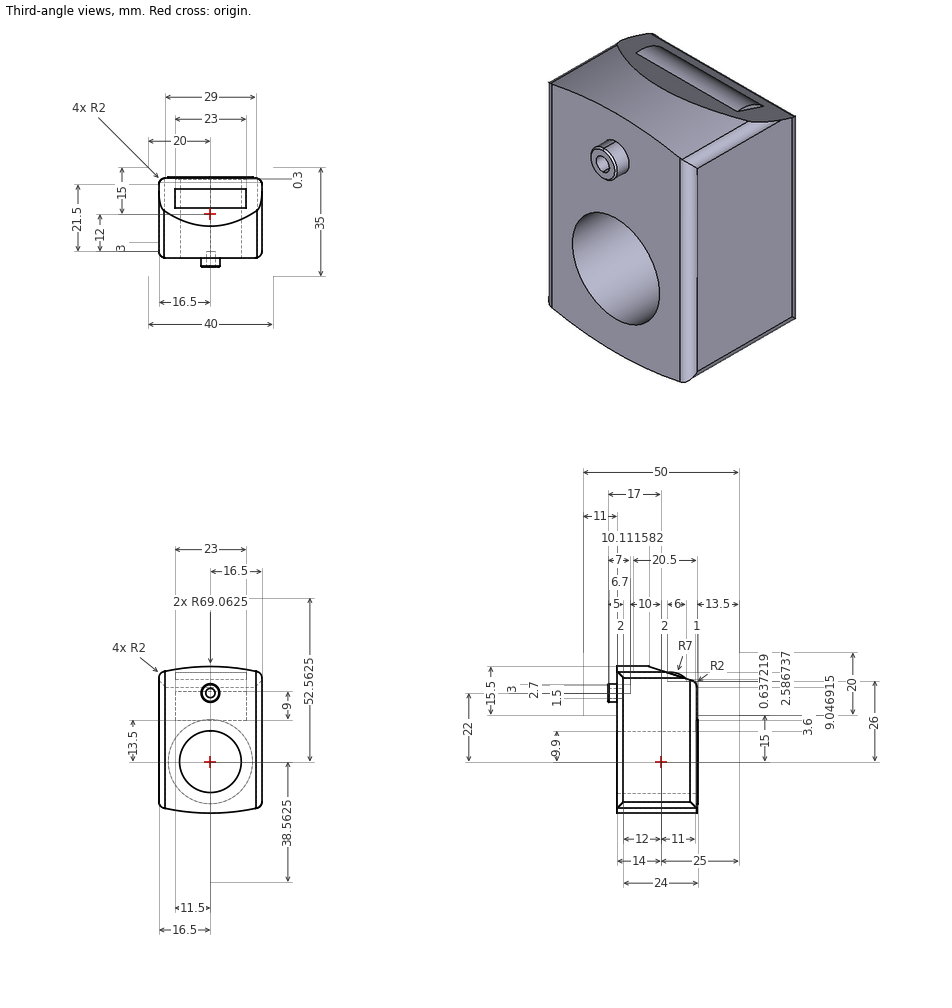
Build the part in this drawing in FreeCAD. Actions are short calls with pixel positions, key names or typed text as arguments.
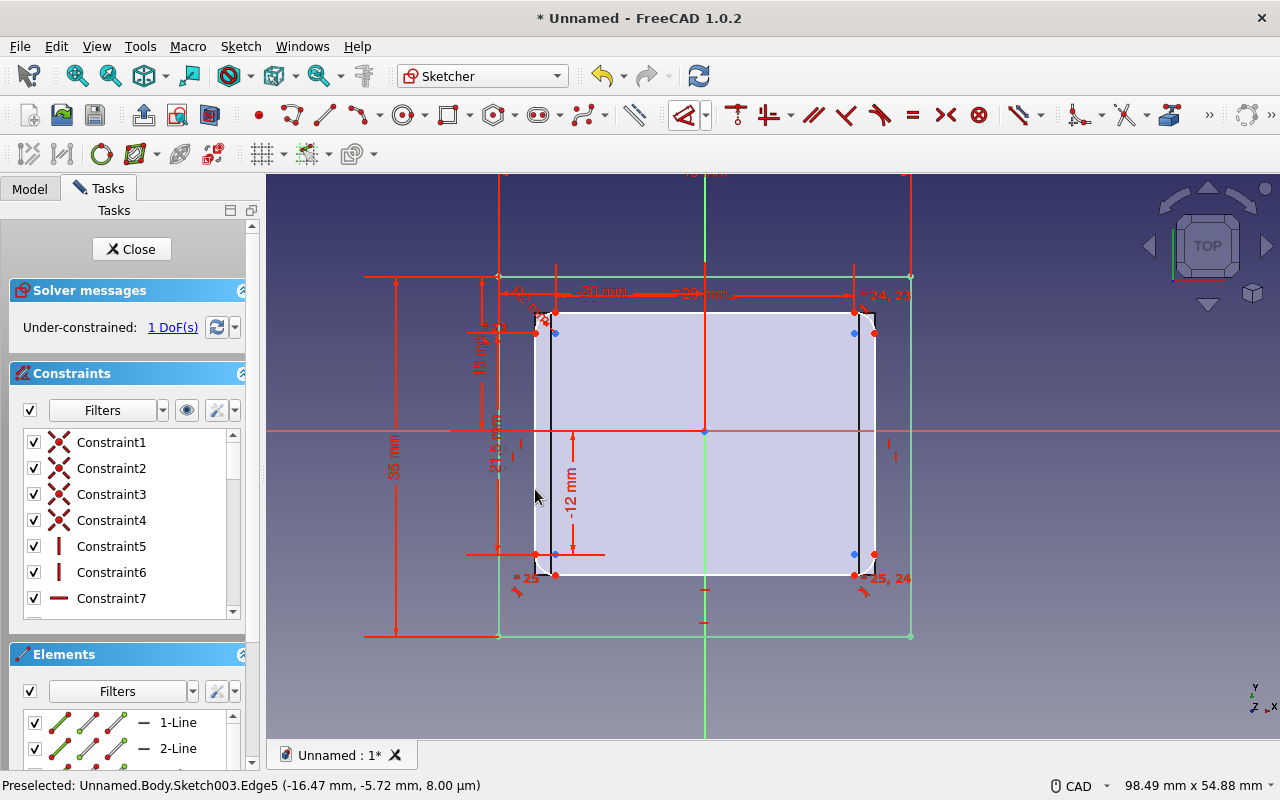
click(535, 555)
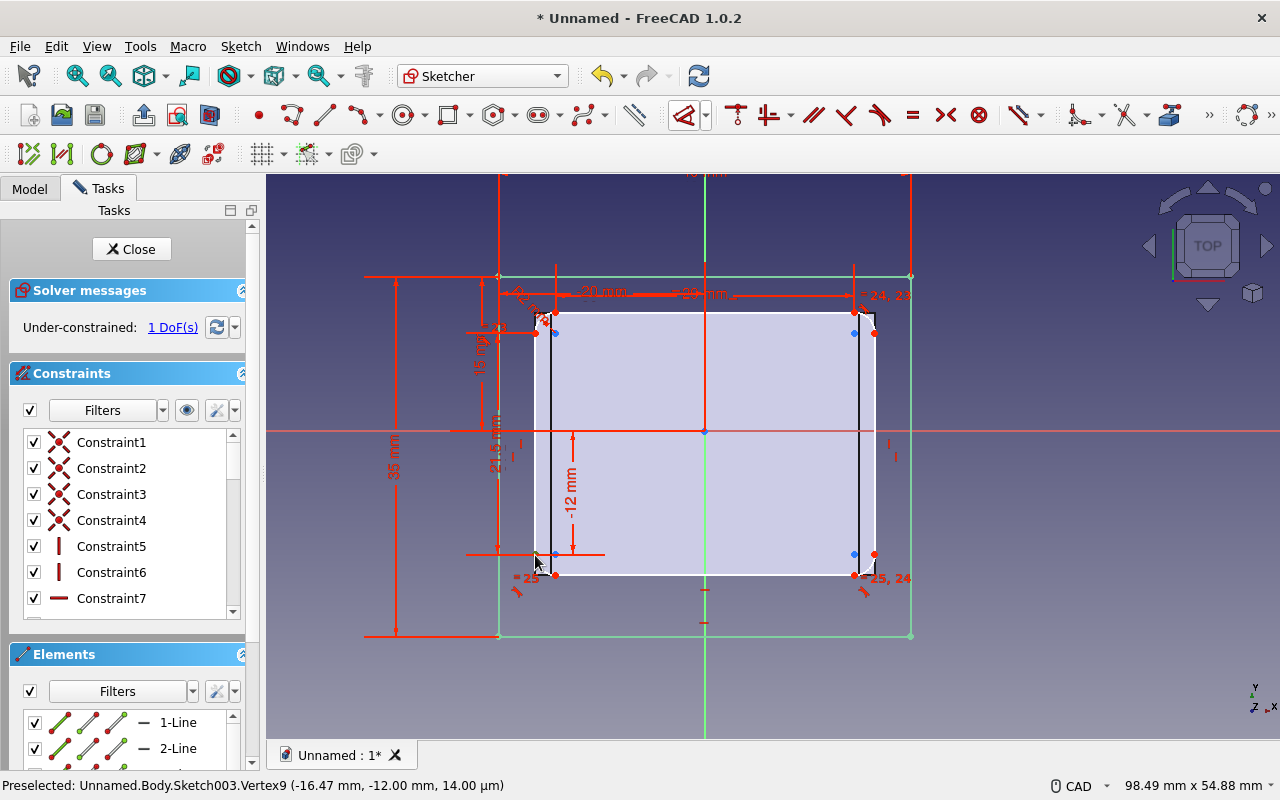
click(706, 116)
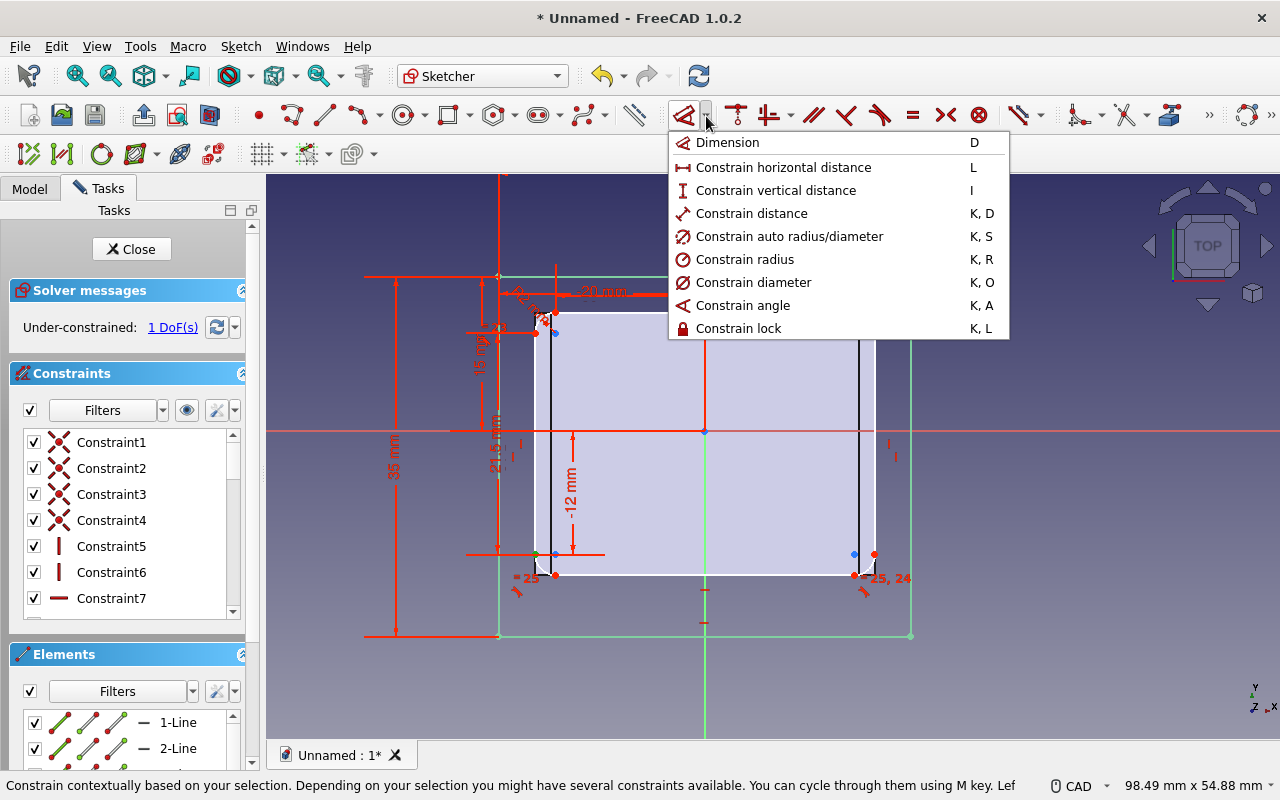
click(839, 168)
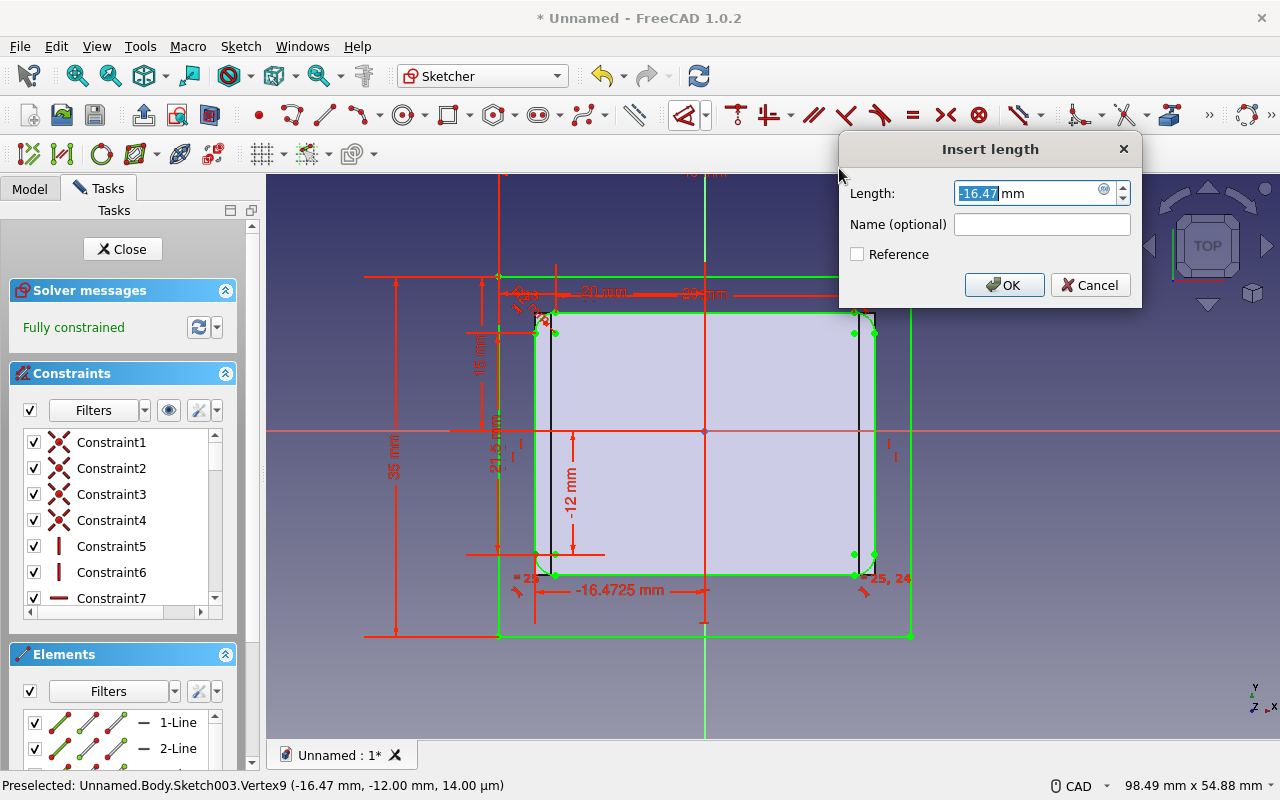
text(-16.5)
key(Return)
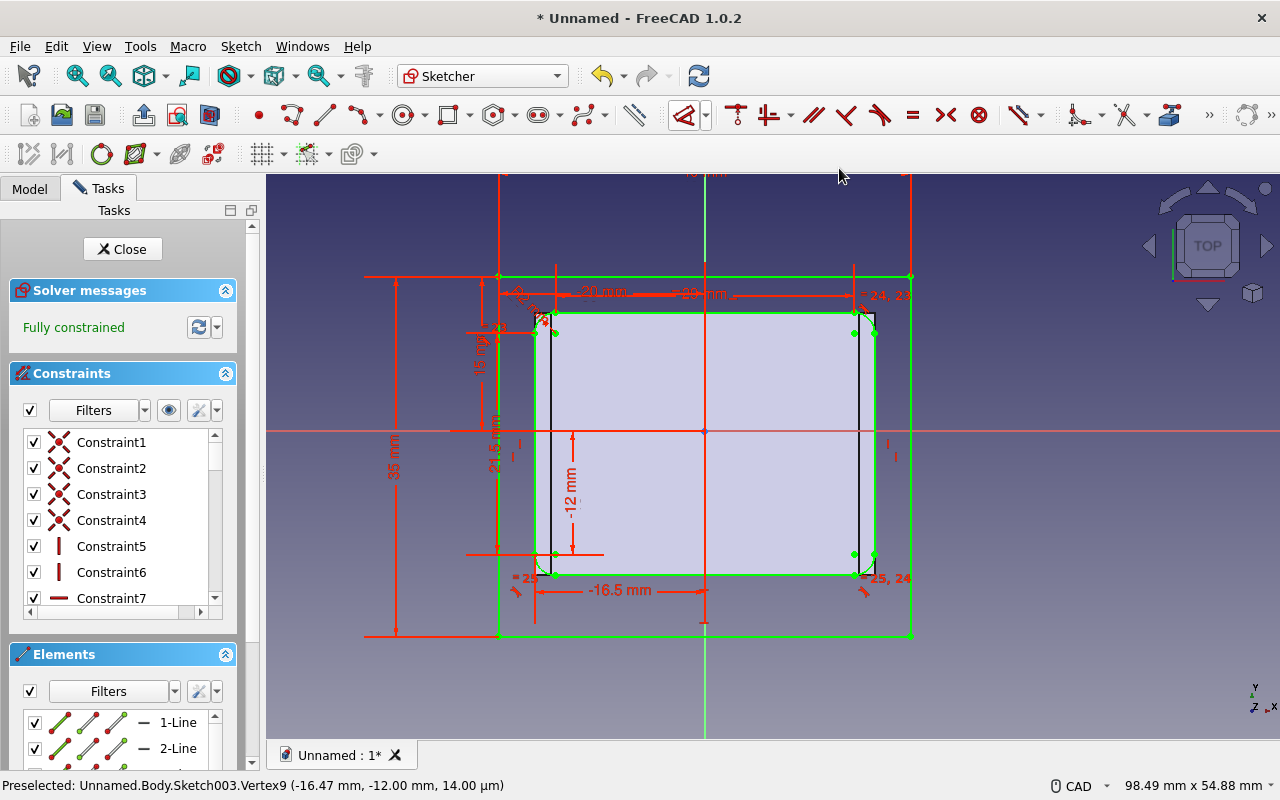
click(123, 249)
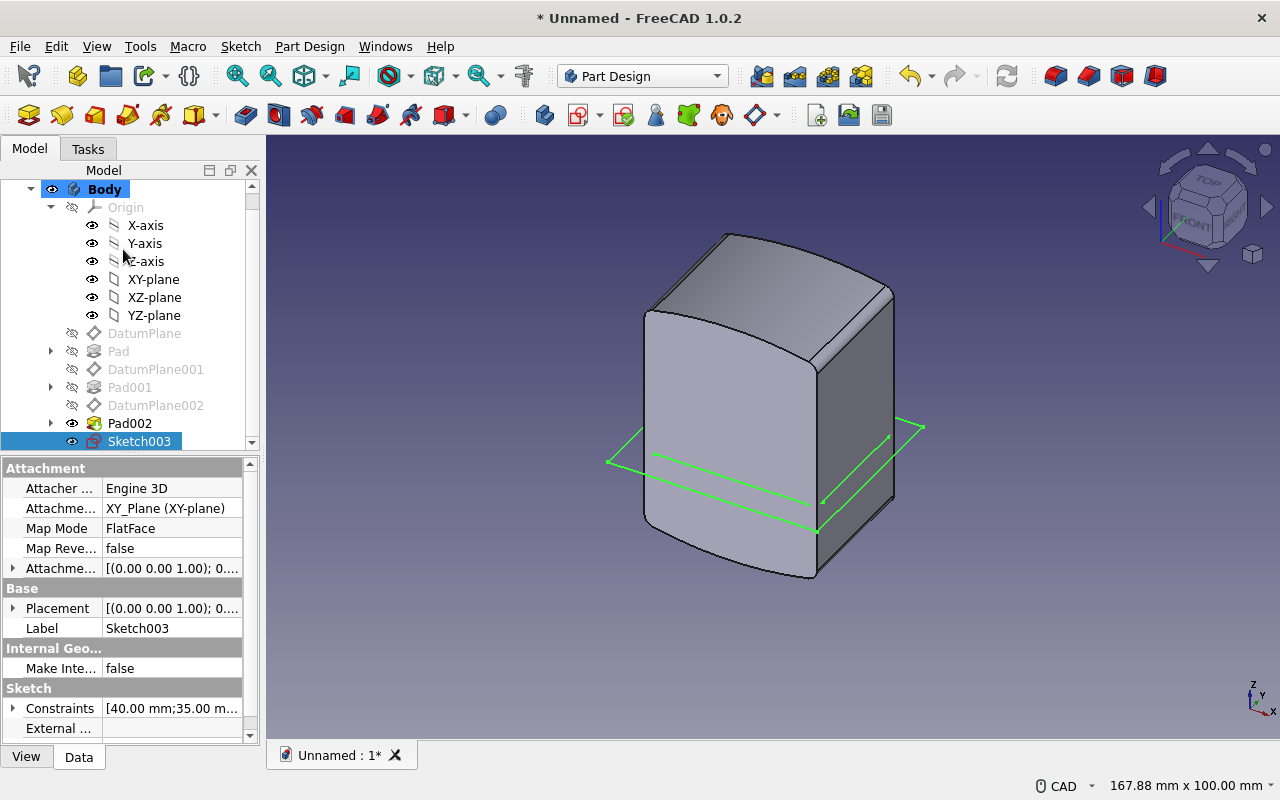
click(246, 116)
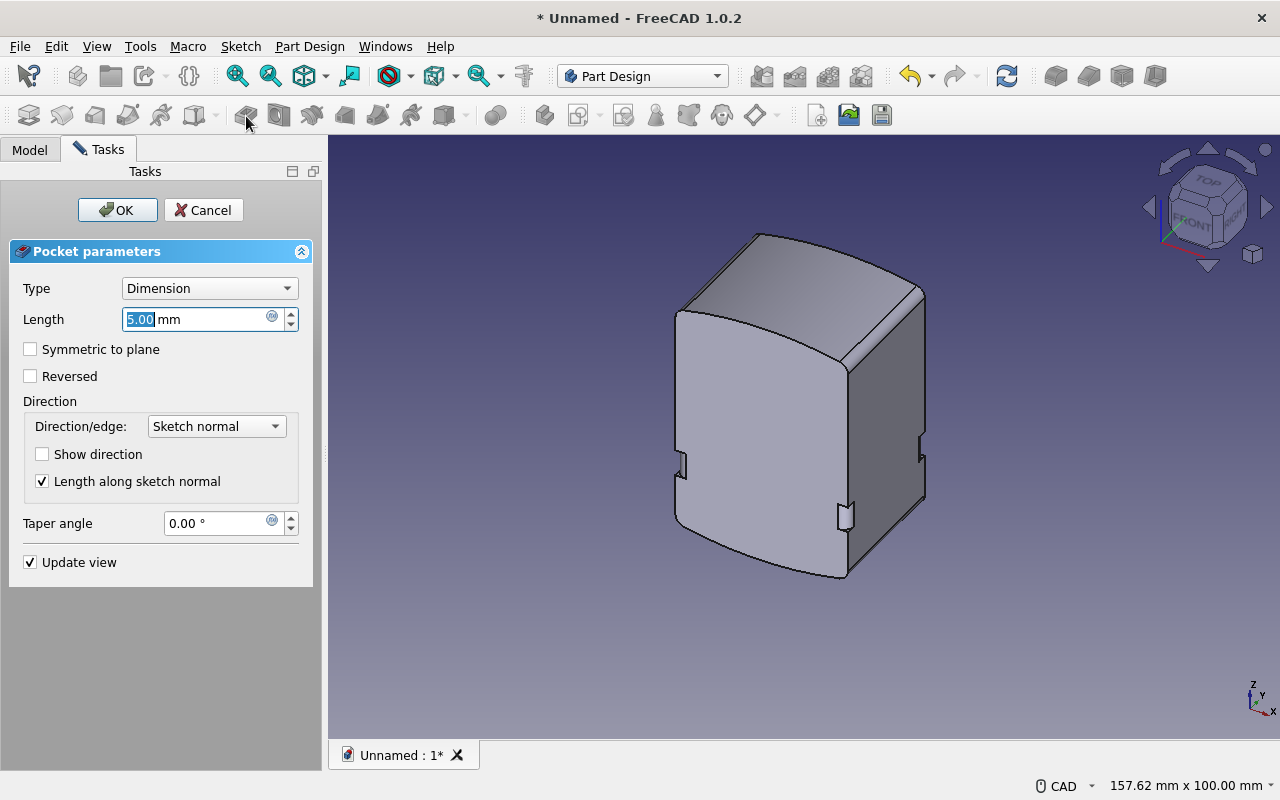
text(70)
key(Tab)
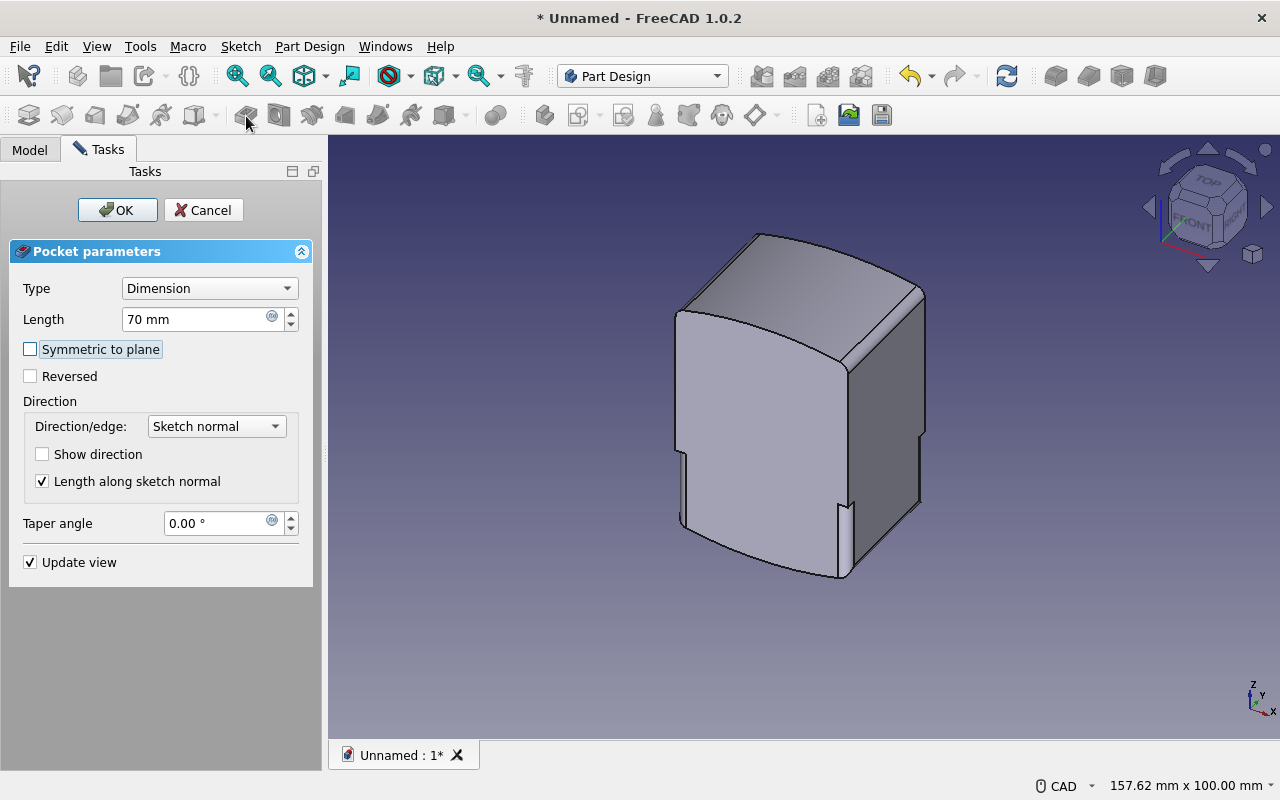
click(31, 349)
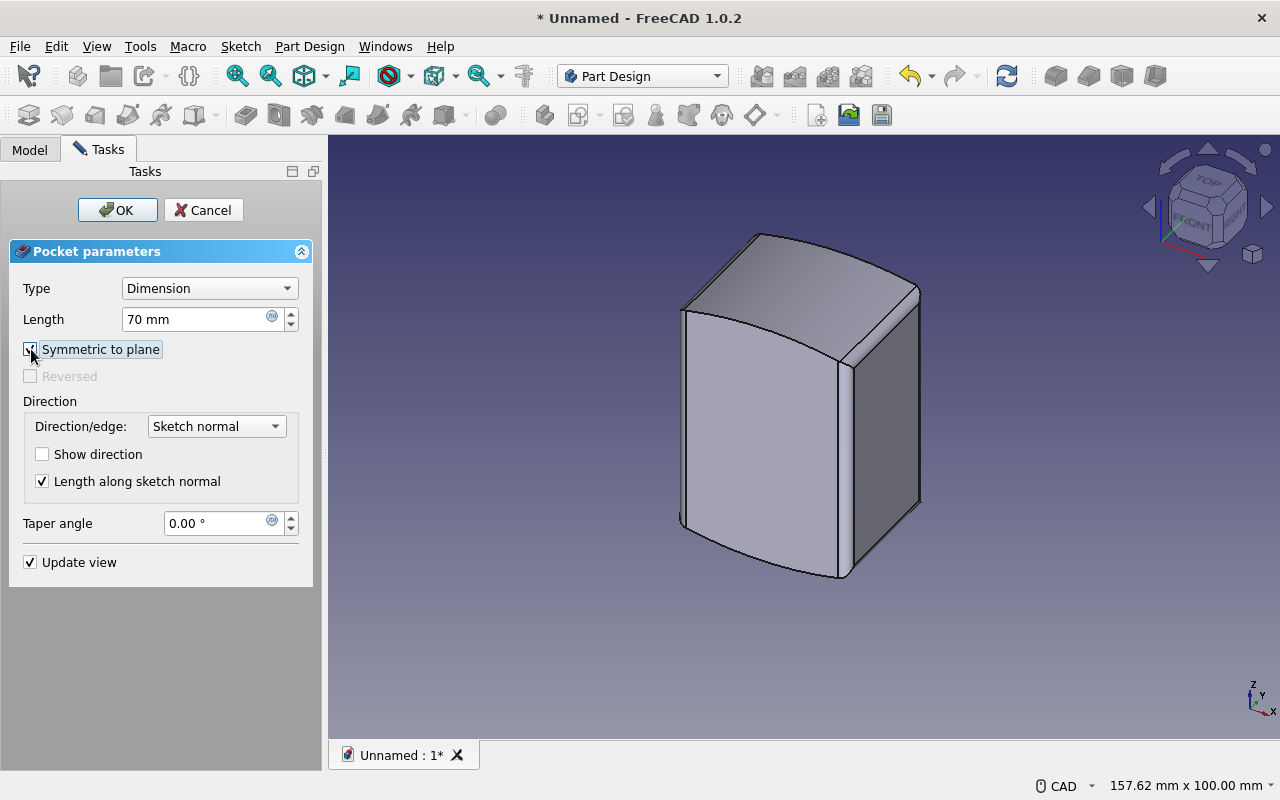
click(118, 210)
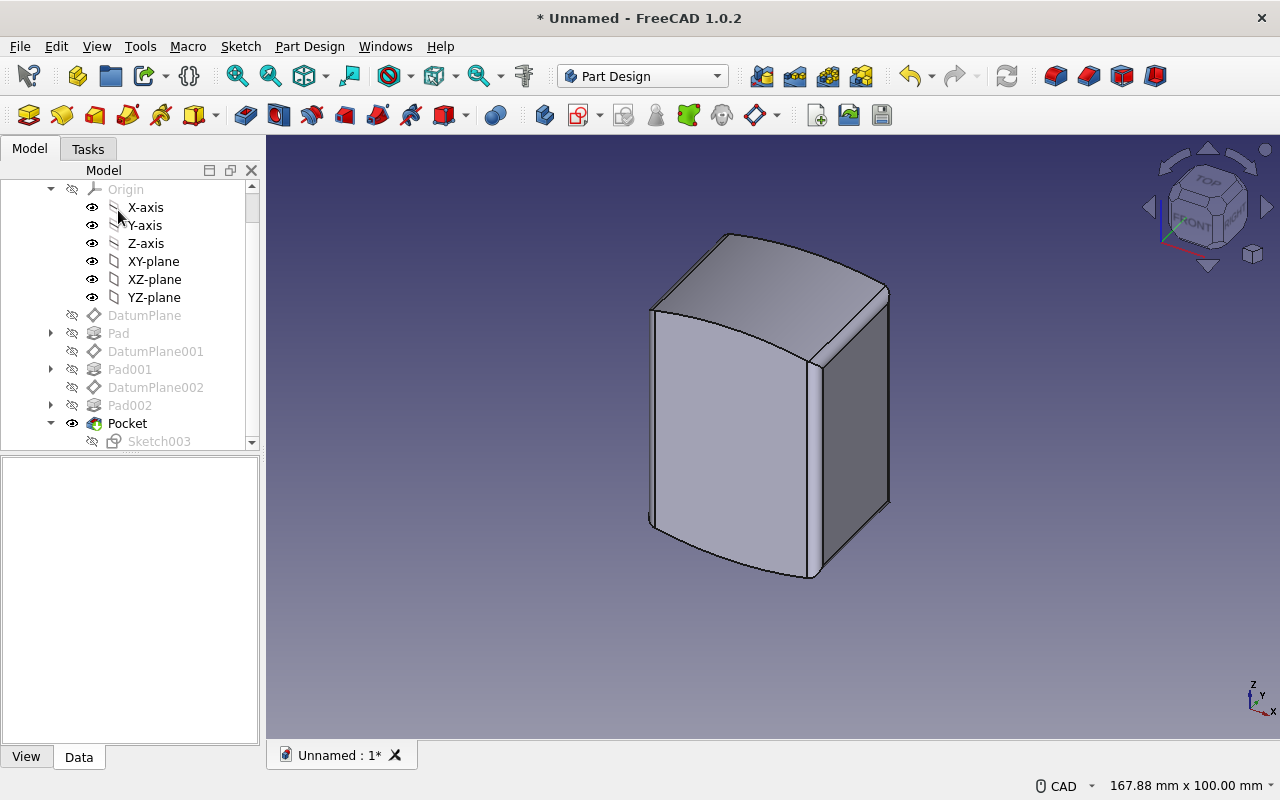
click(578, 116)